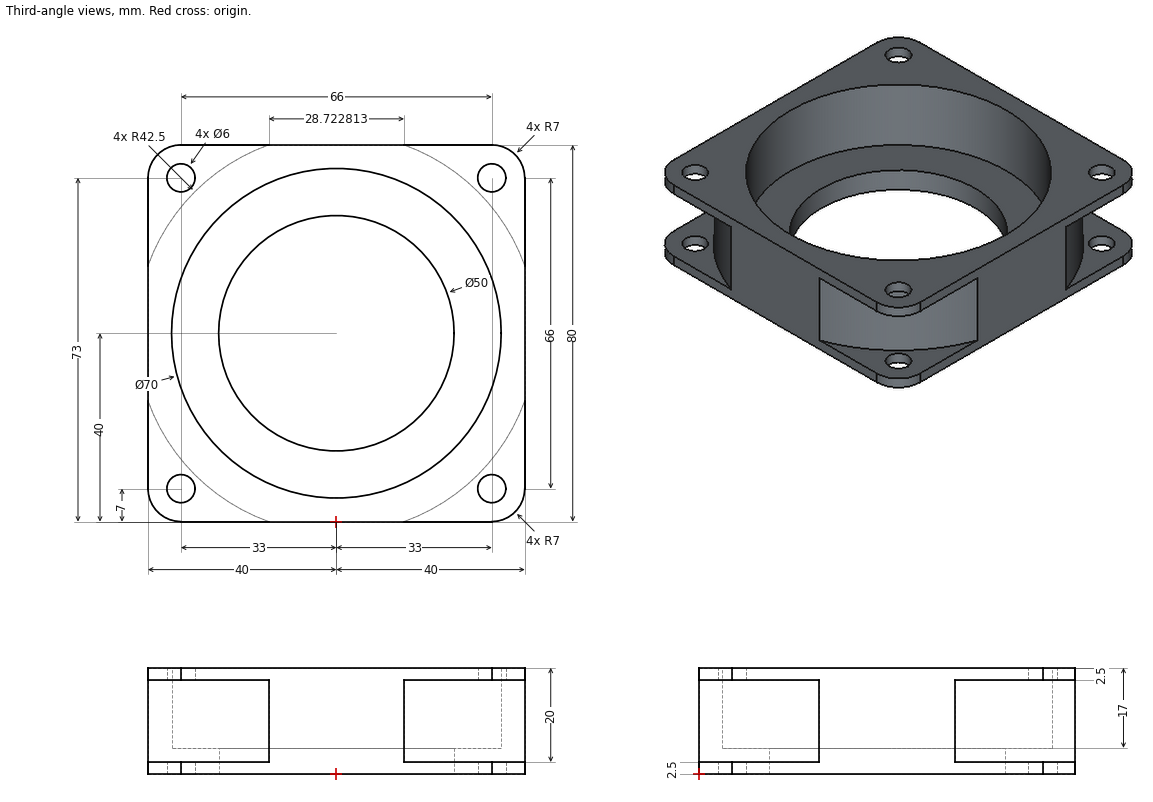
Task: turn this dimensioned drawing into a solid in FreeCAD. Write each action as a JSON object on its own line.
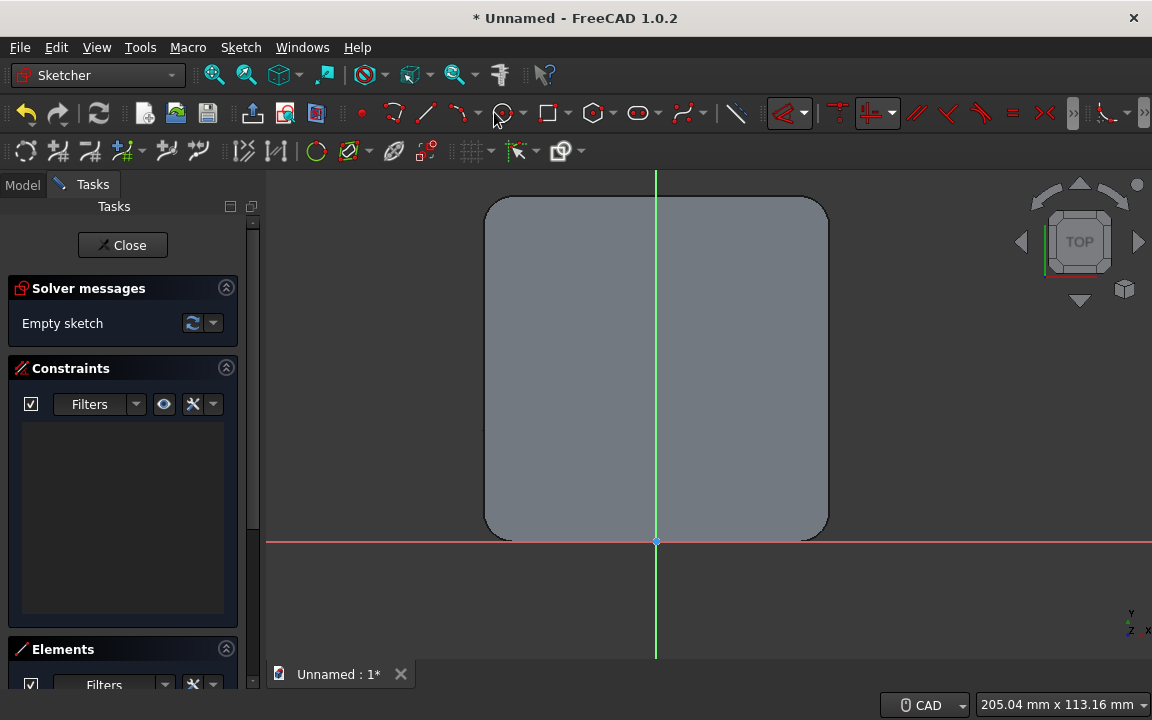
{"action": "scroll", "coordinate": [568, 572], "scroll_direction": "down", "scroll_amount": 1}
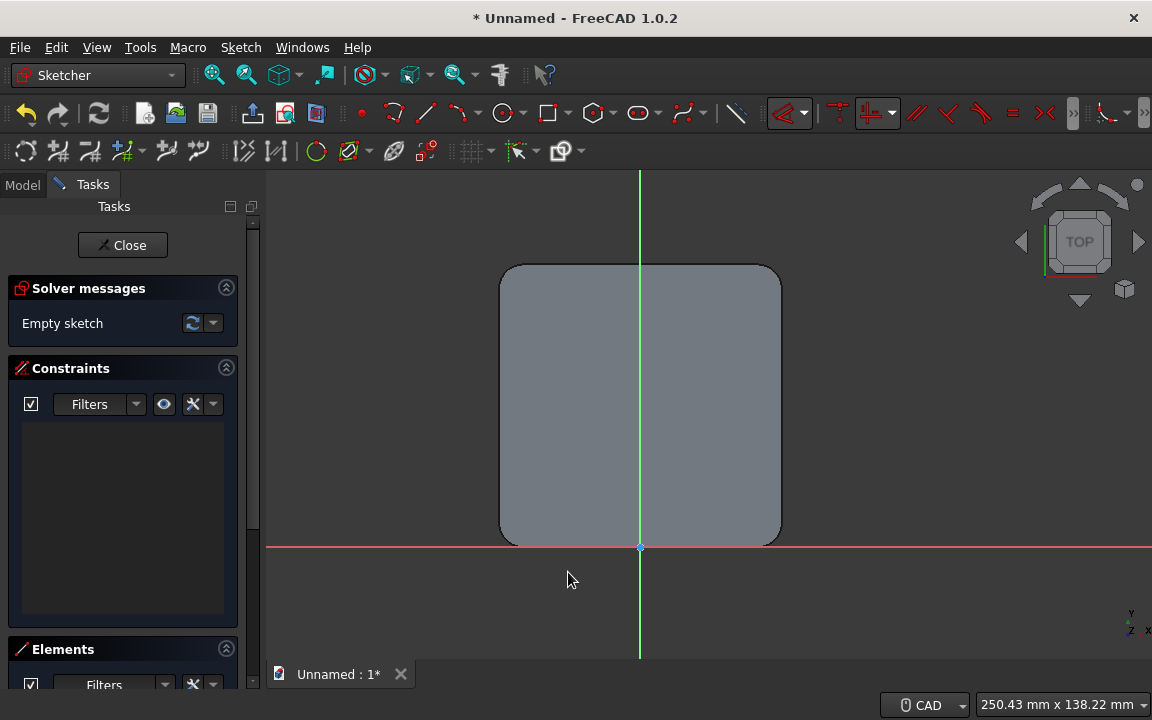
{"action": "key", "text": "g c"}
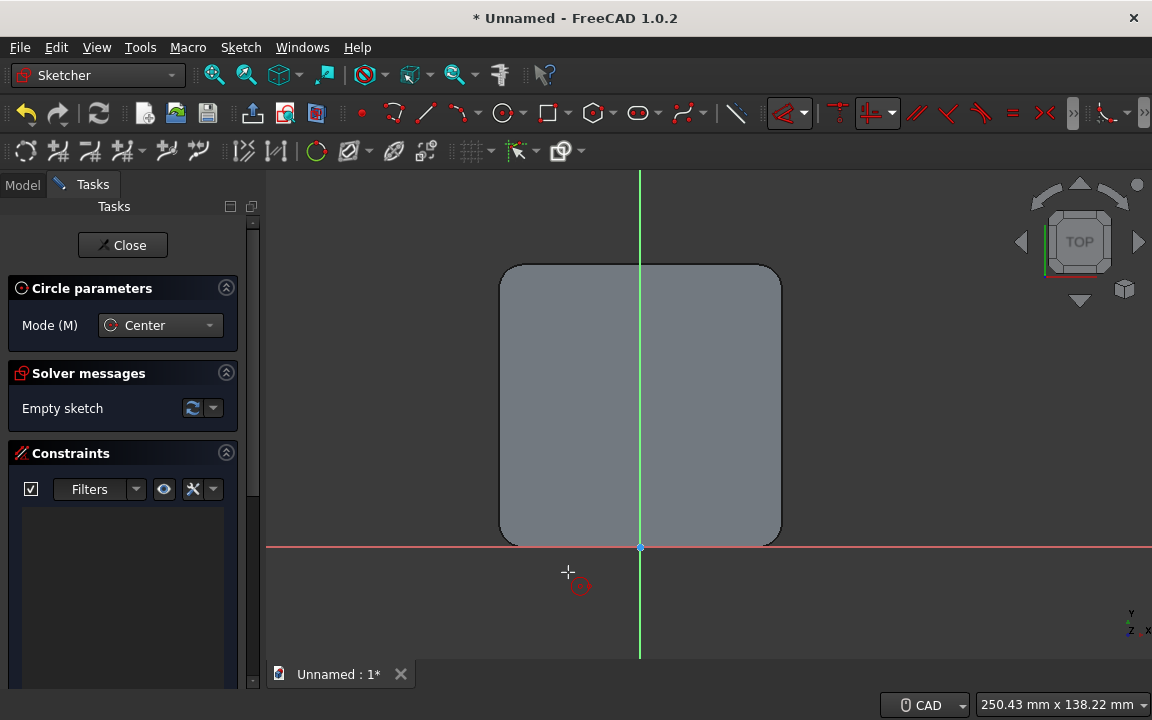
{"action": "left_click", "coordinate": [640, 406]}
{"action": "mouse_move", "coordinate": [728, 318]}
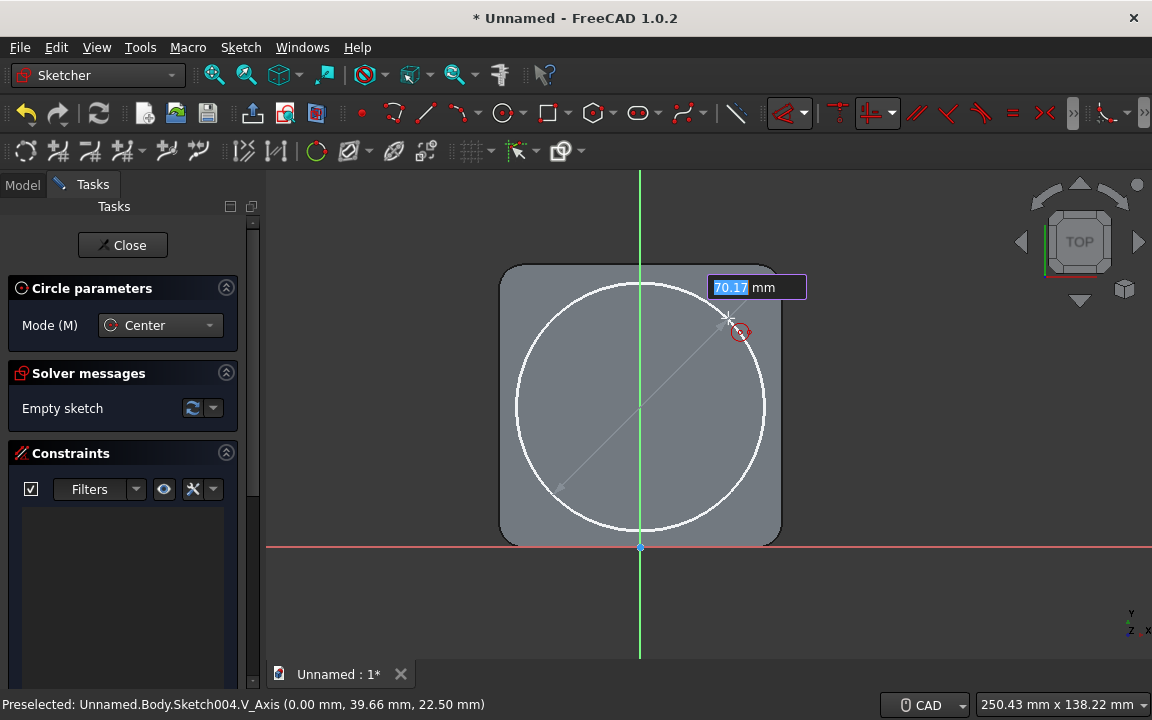
{"action": "type", "text": "70"}
{"action": "key", "text": "Return"}
{"action": "key", "text": "Escape"}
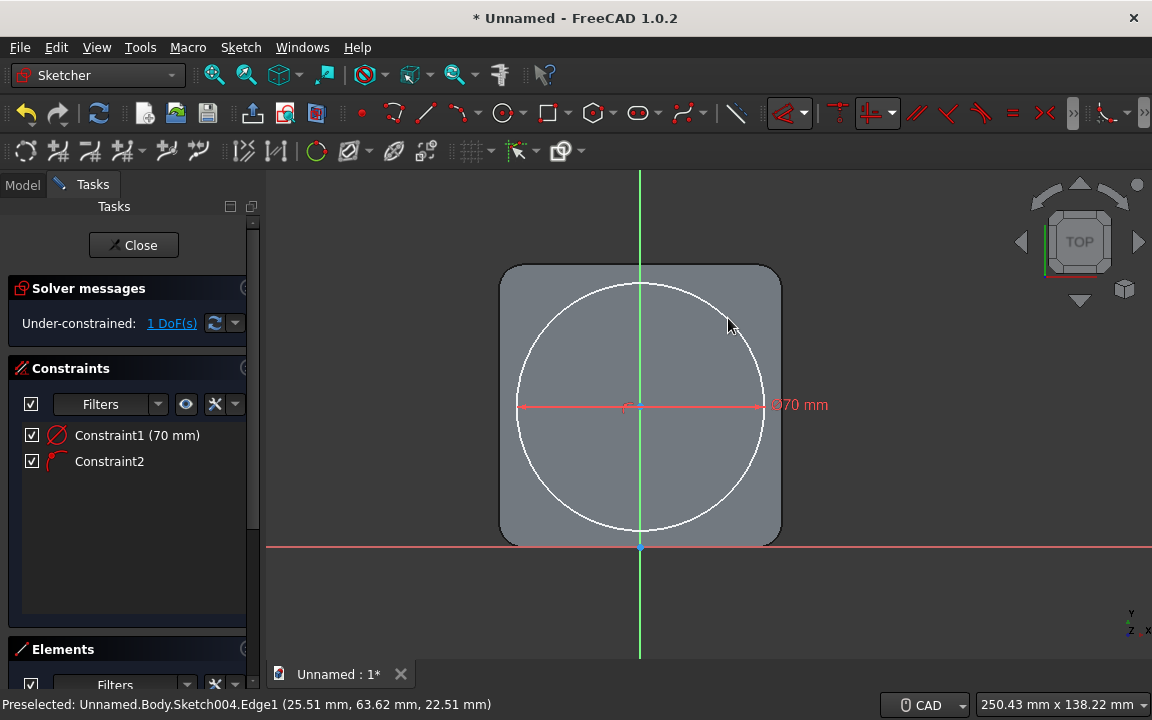
{"action": "key", "text": "d"}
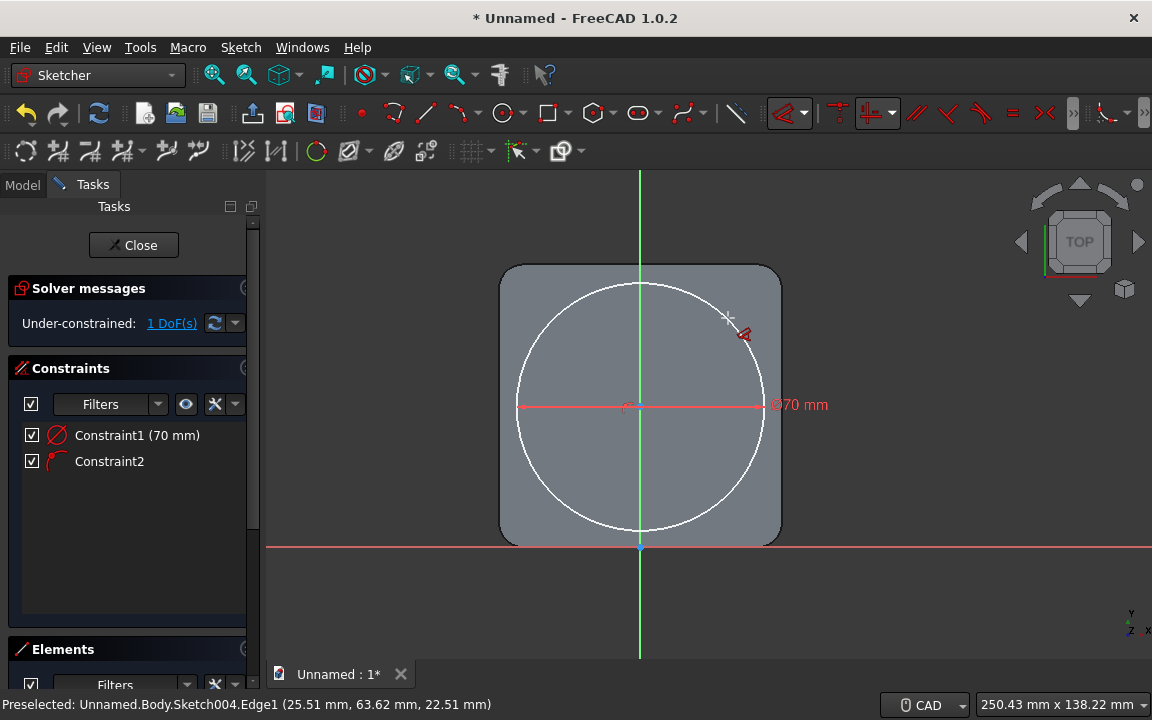
{"action": "left_click", "coordinate": [640, 407]}
{"action": "left_click", "coordinate": [674, 477]}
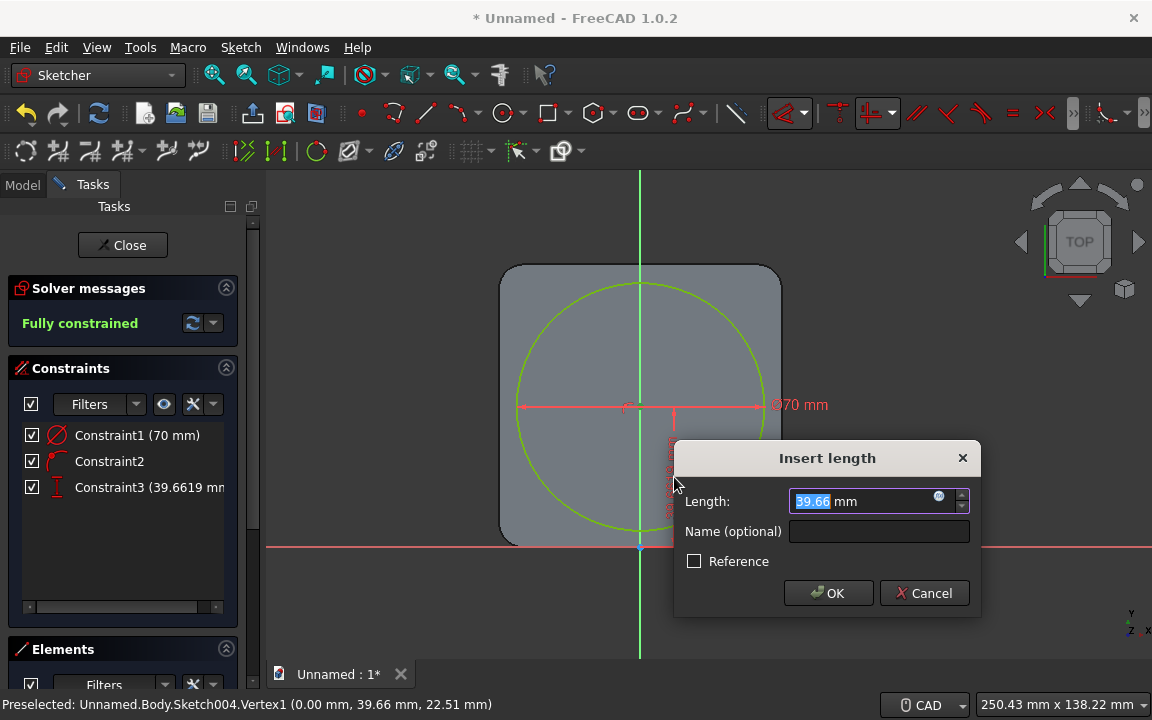
{"action": "type", "text": "40"}
{"action": "key", "text": "Return"}
{"action": "key", "text": "Escape"}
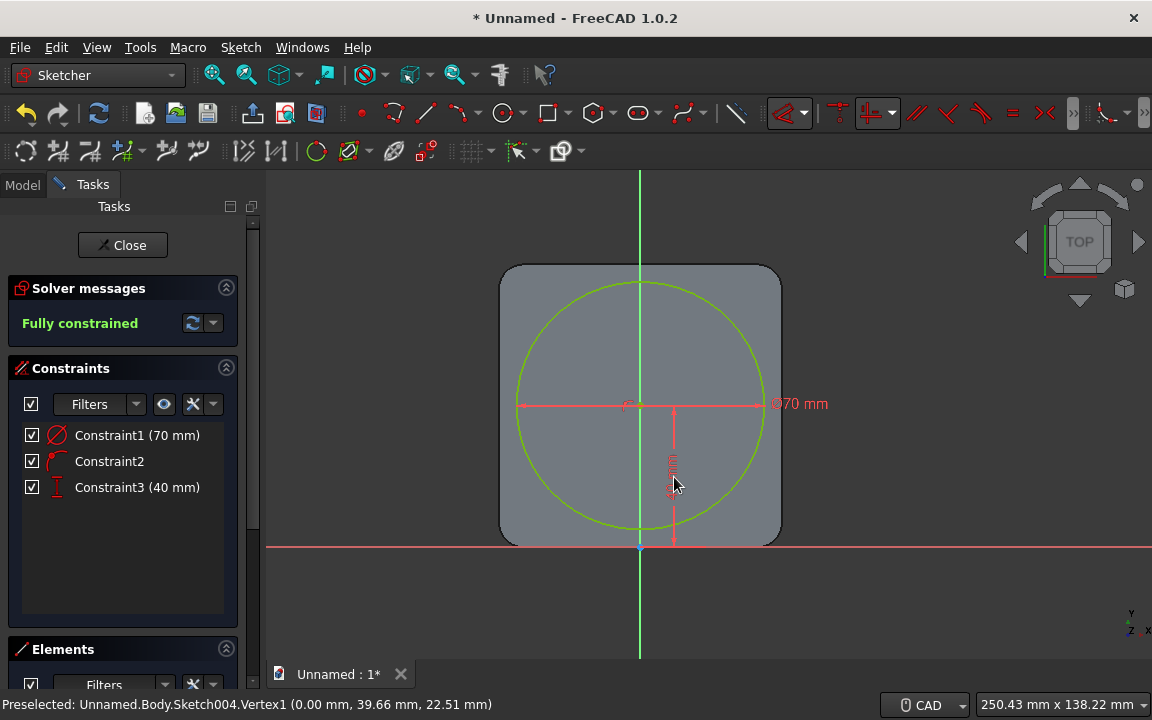
{"action": "left_click", "coordinate": [123, 245]}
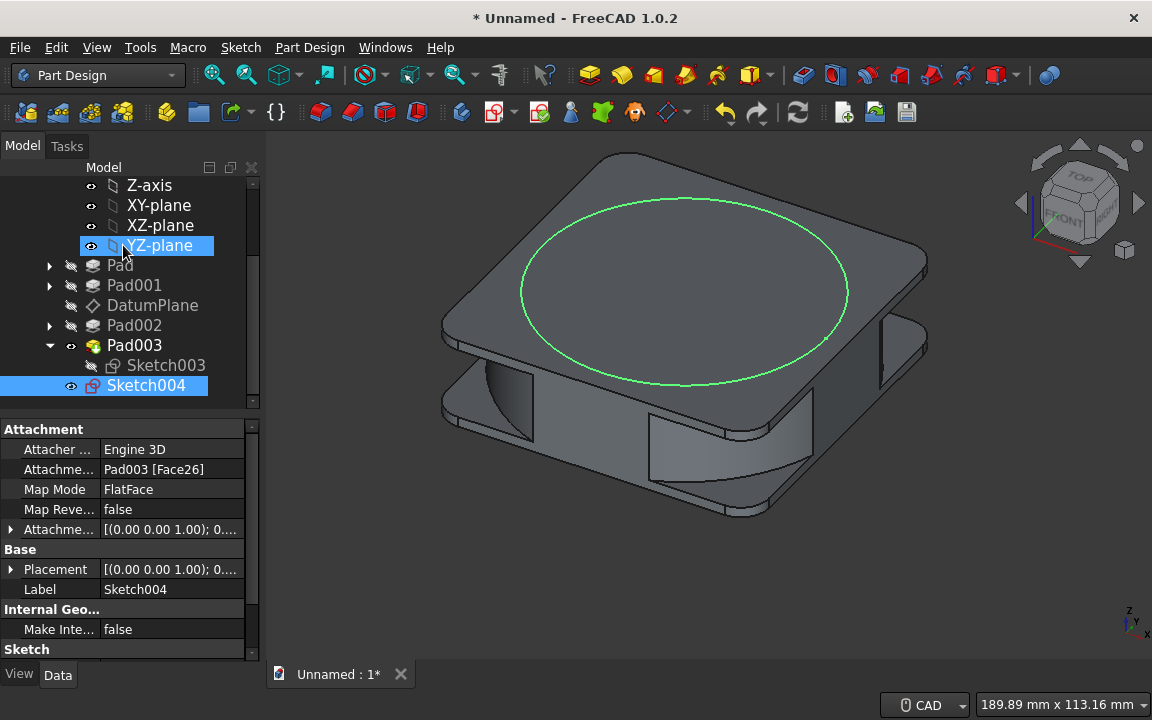
{"action": "left_click", "coordinate": [804, 76]}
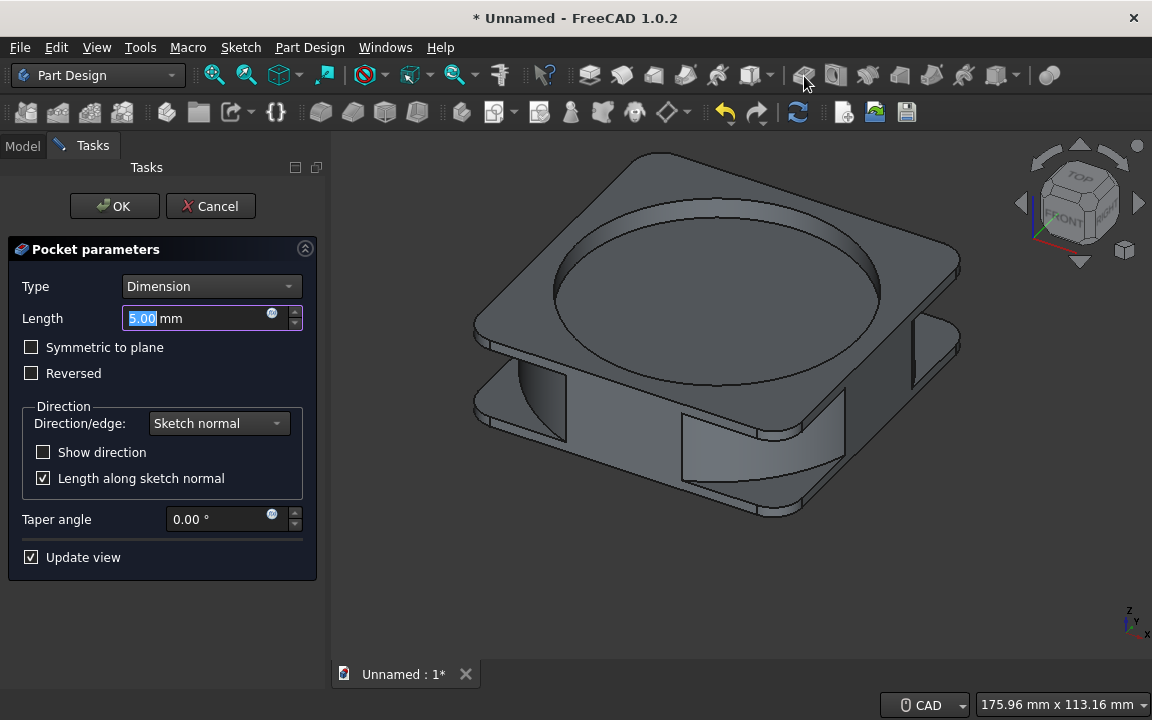
{"action": "type", "text": "17"}
{"action": "key", "text": "Tab"}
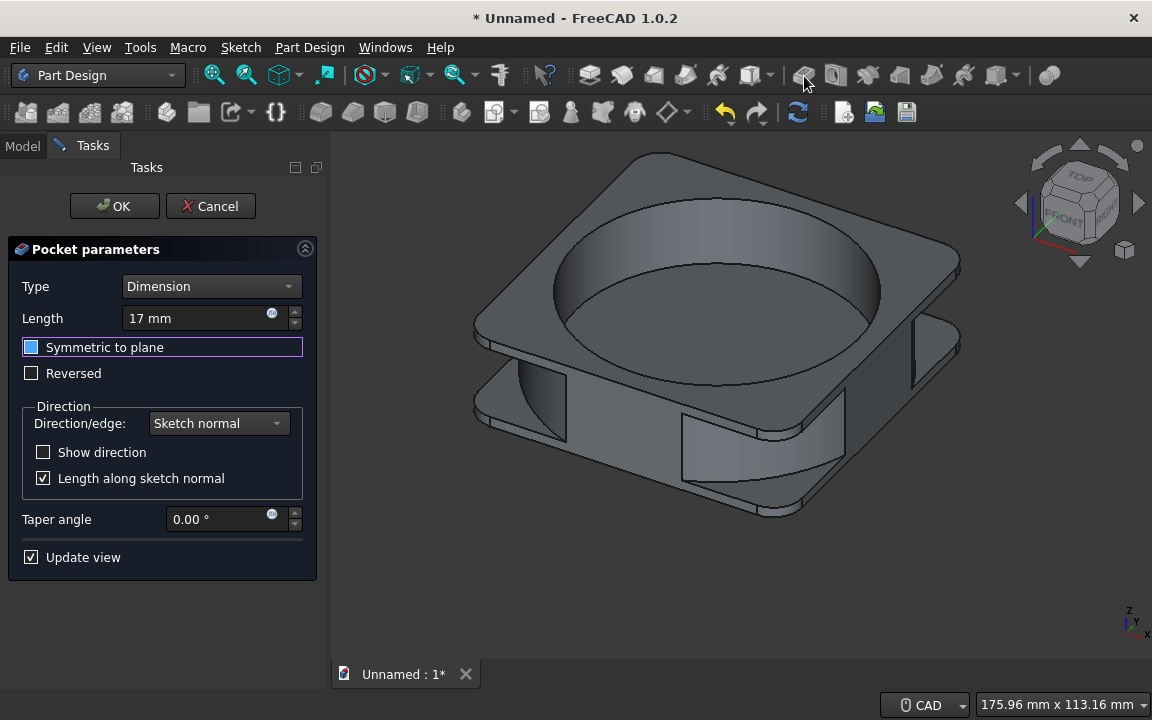
{"action": "left_click", "coordinate": [115, 206]}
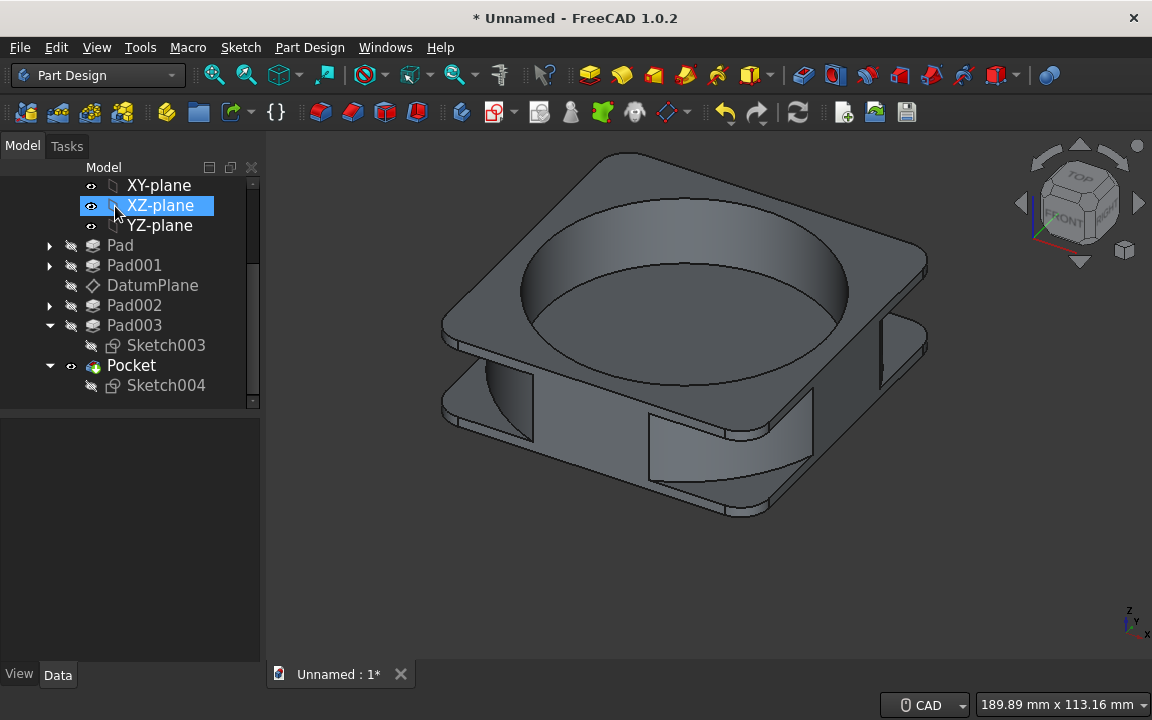
{"action": "left_click", "coordinate": [685, 356]}